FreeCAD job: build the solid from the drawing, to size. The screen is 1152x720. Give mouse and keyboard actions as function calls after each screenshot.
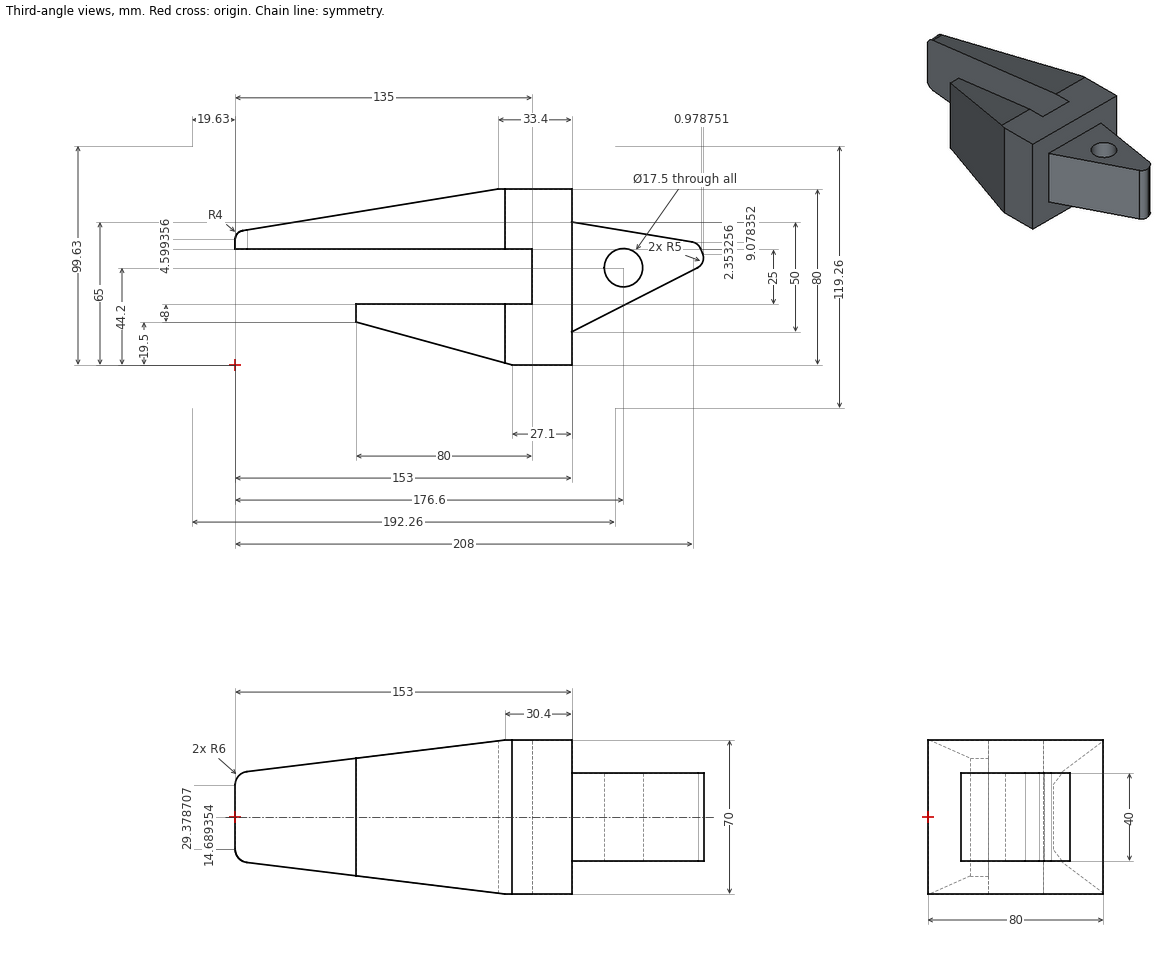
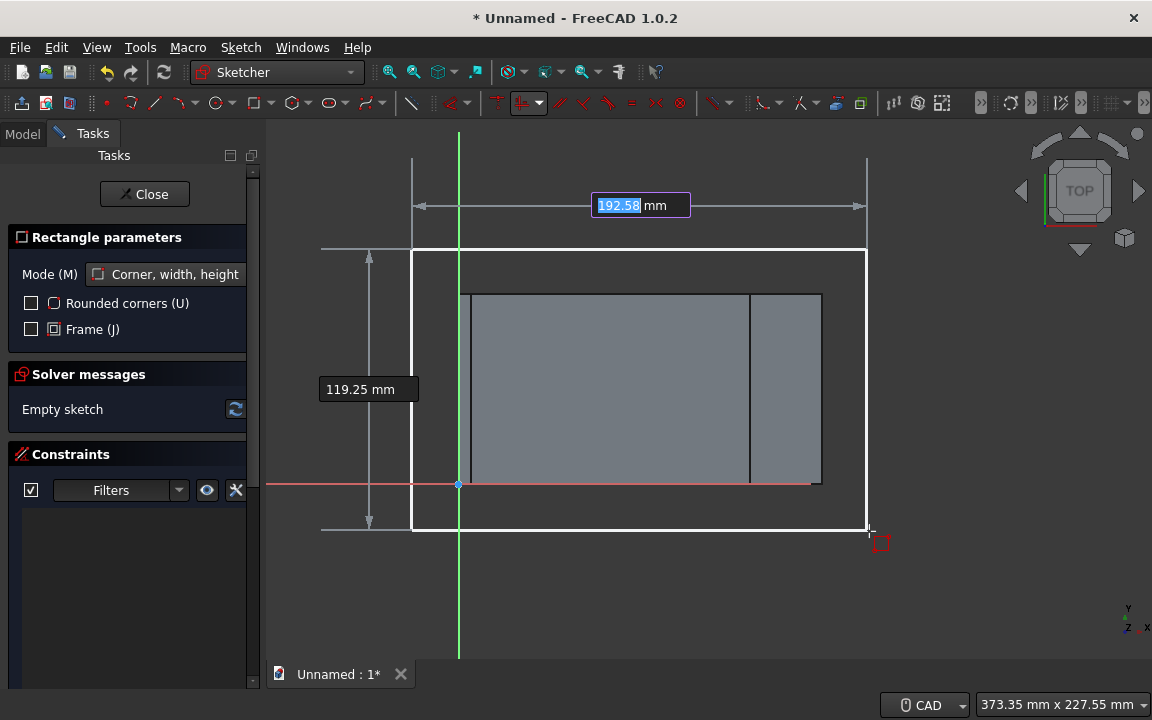
text(192.26)
key(Tab)
text(119.26)
key(Return)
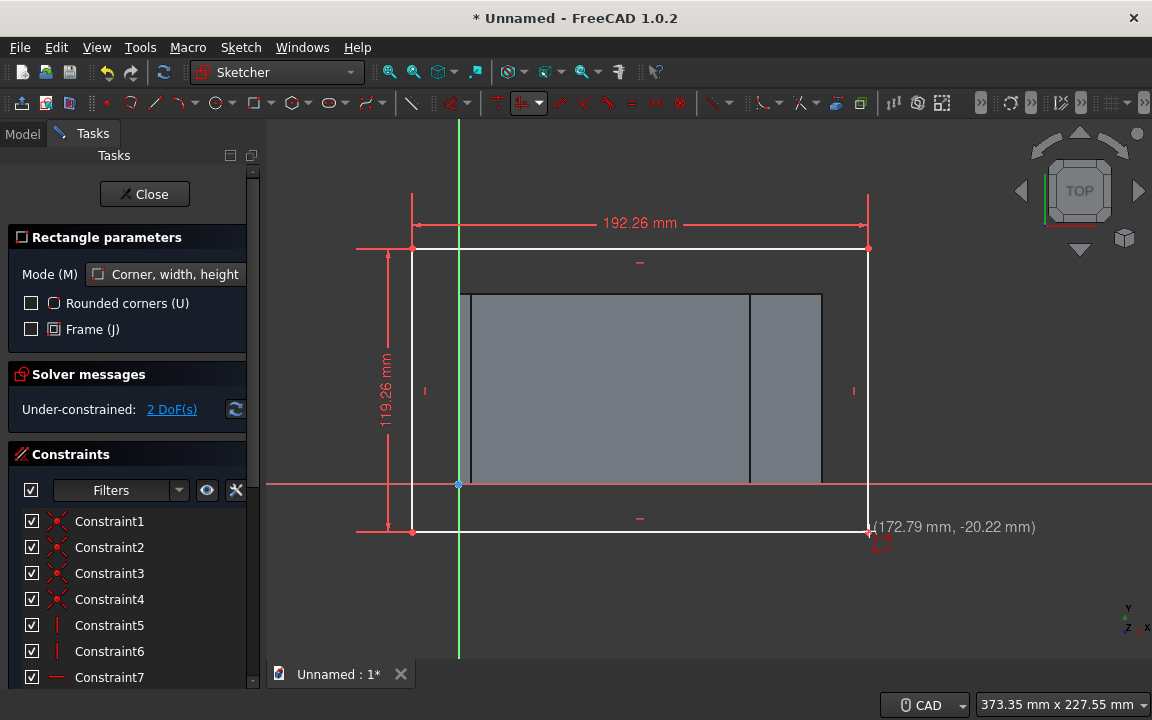
click(132, 104)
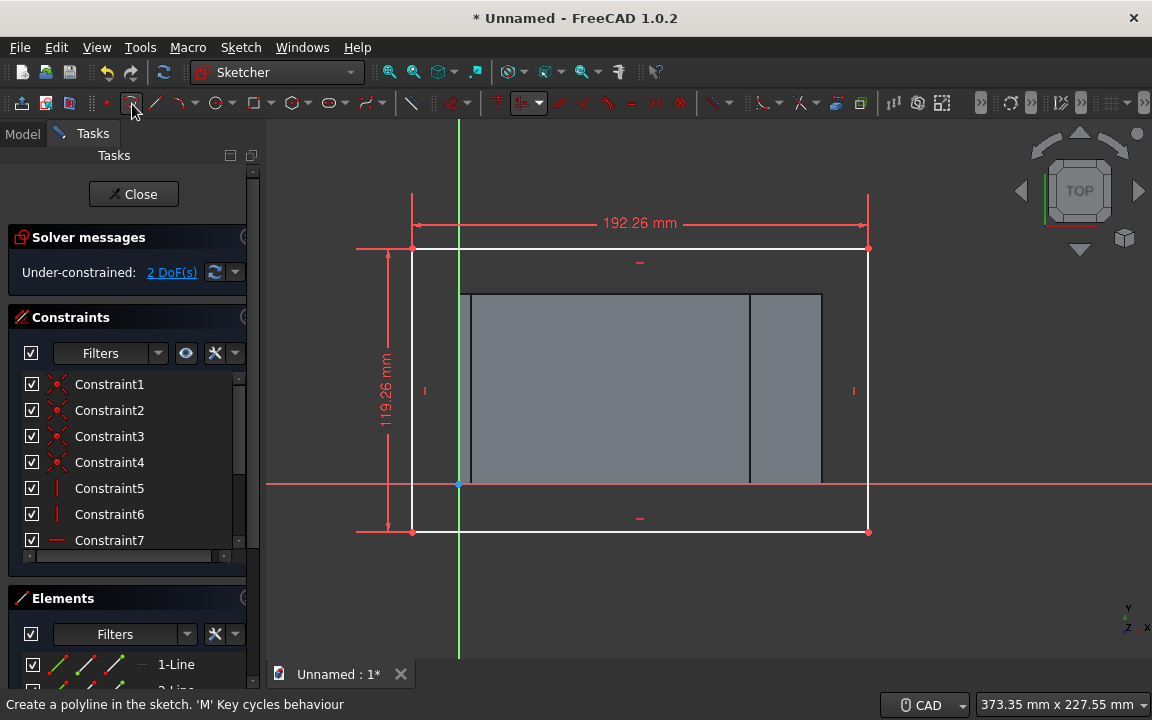
scroll(467, 339, up, 4)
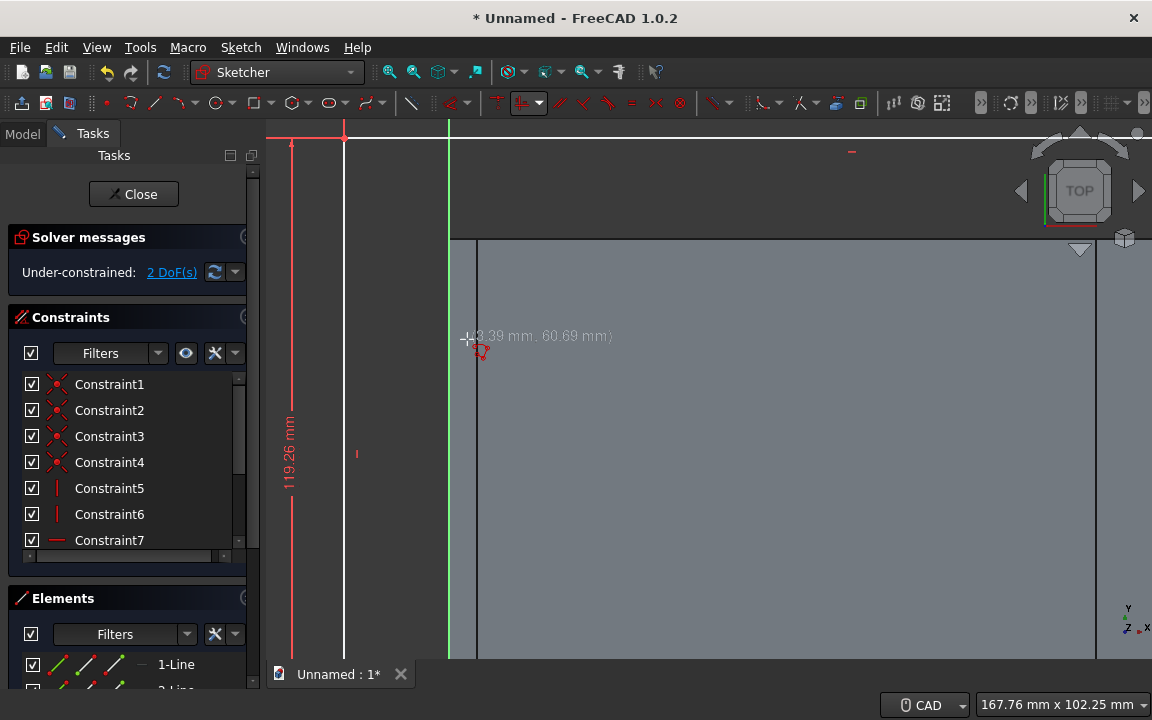
click(467, 339)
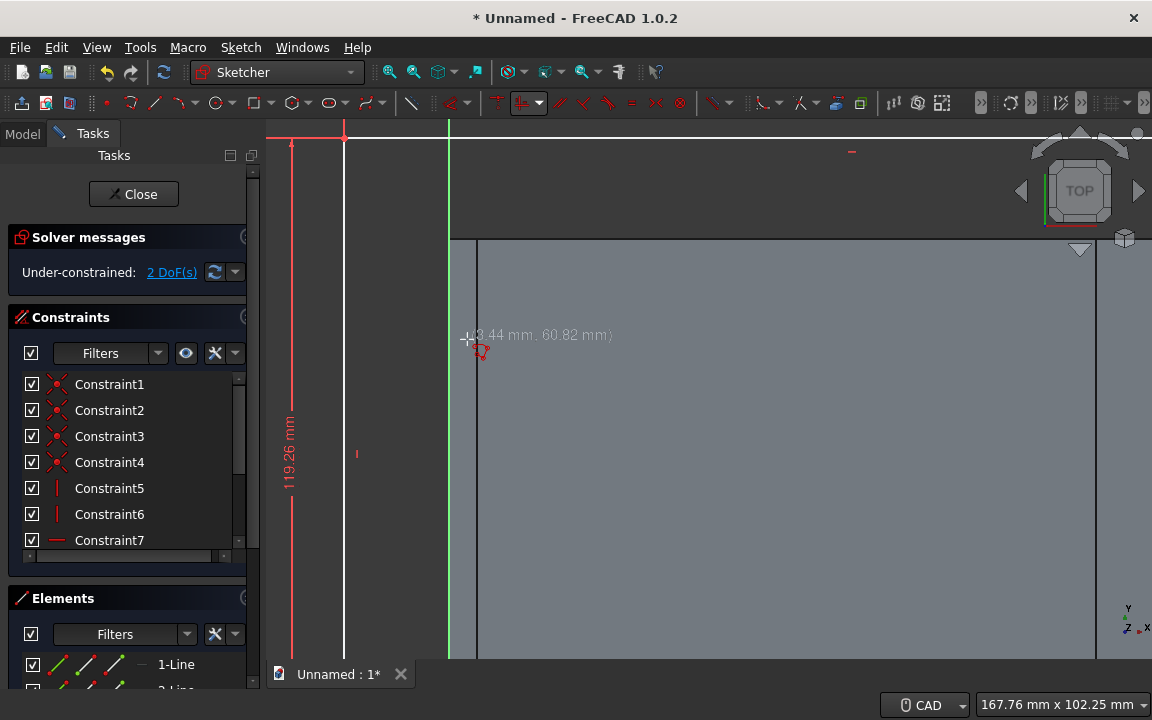
scroll(467, 339, down, 4)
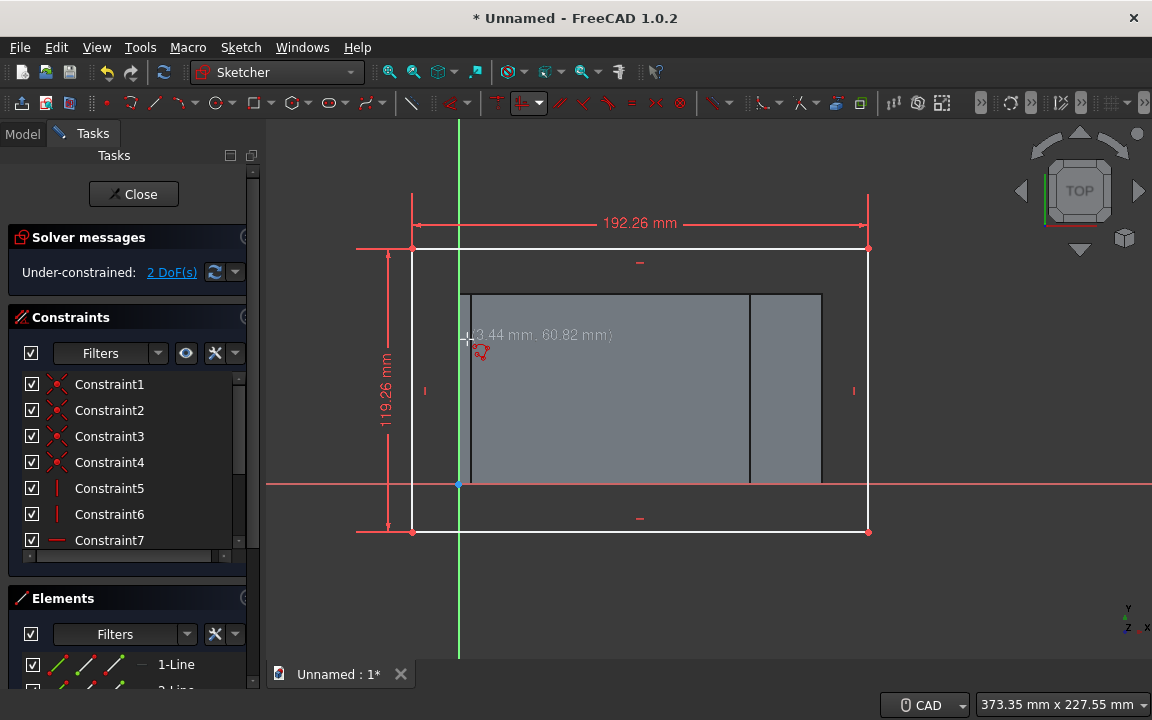
click(743, 294)
click(822, 294)
click(822, 484)
click(758, 475)
click(589, 438)
click(589, 419)
click(779, 419)
click(779, 359)
click(459, 359)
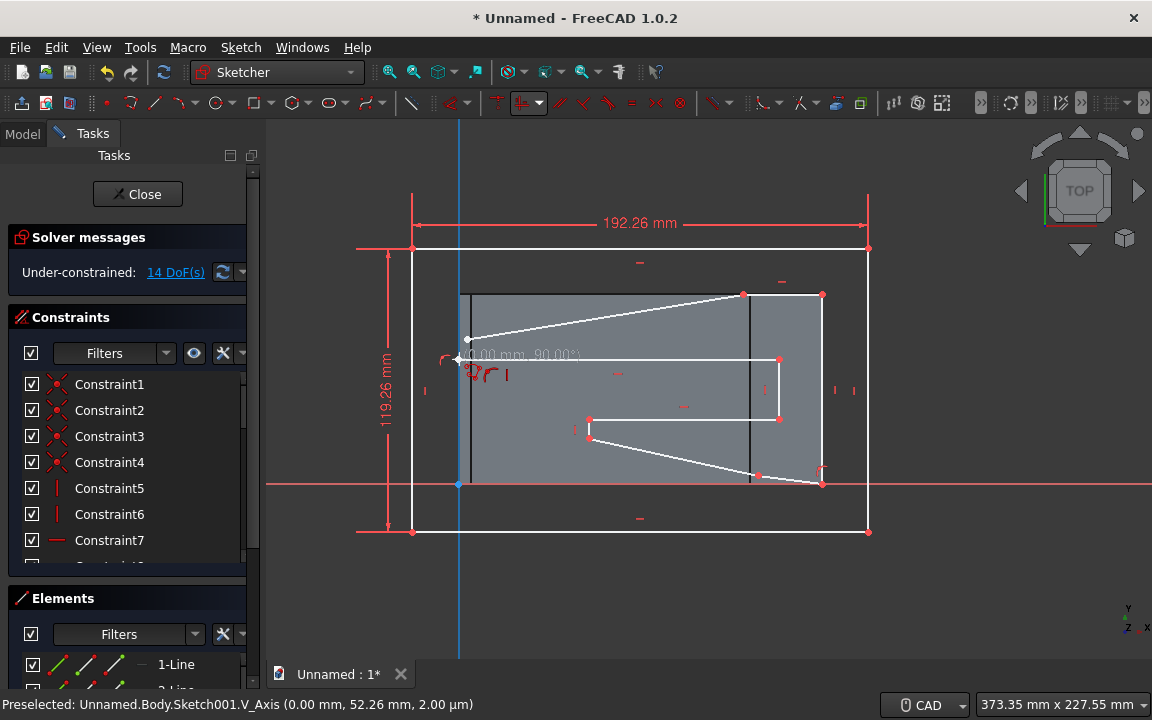
scroll(459, 349, up, 2)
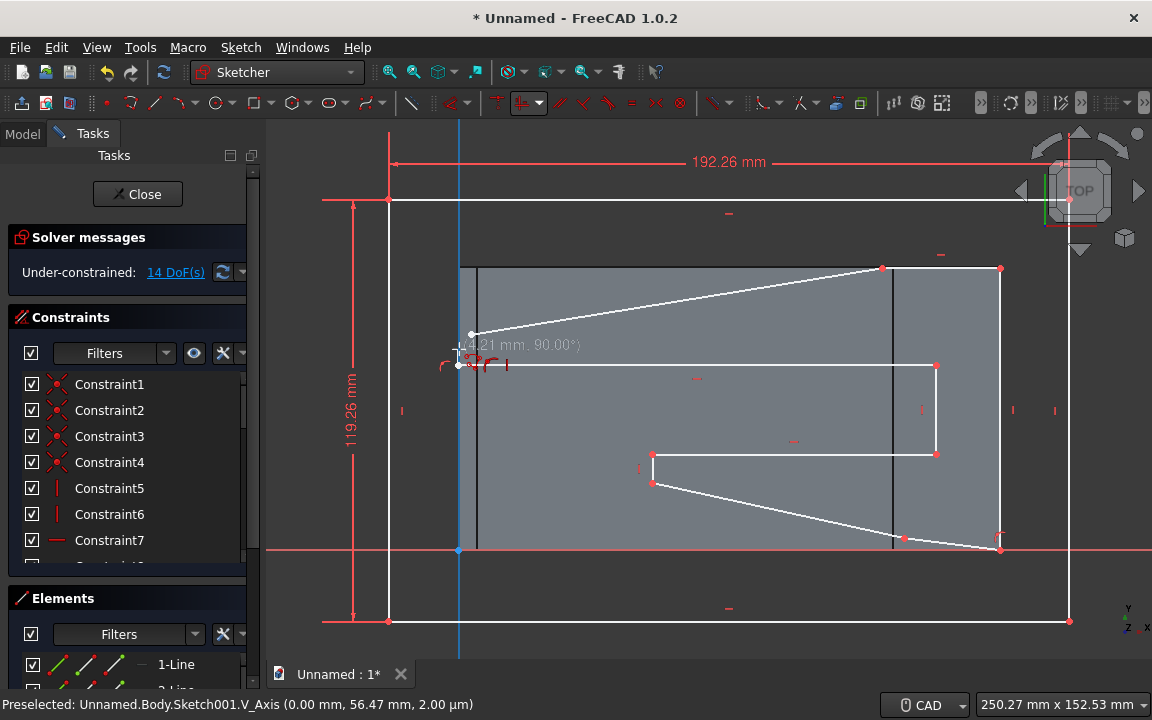
click(468, 348)
right_click(468, 348)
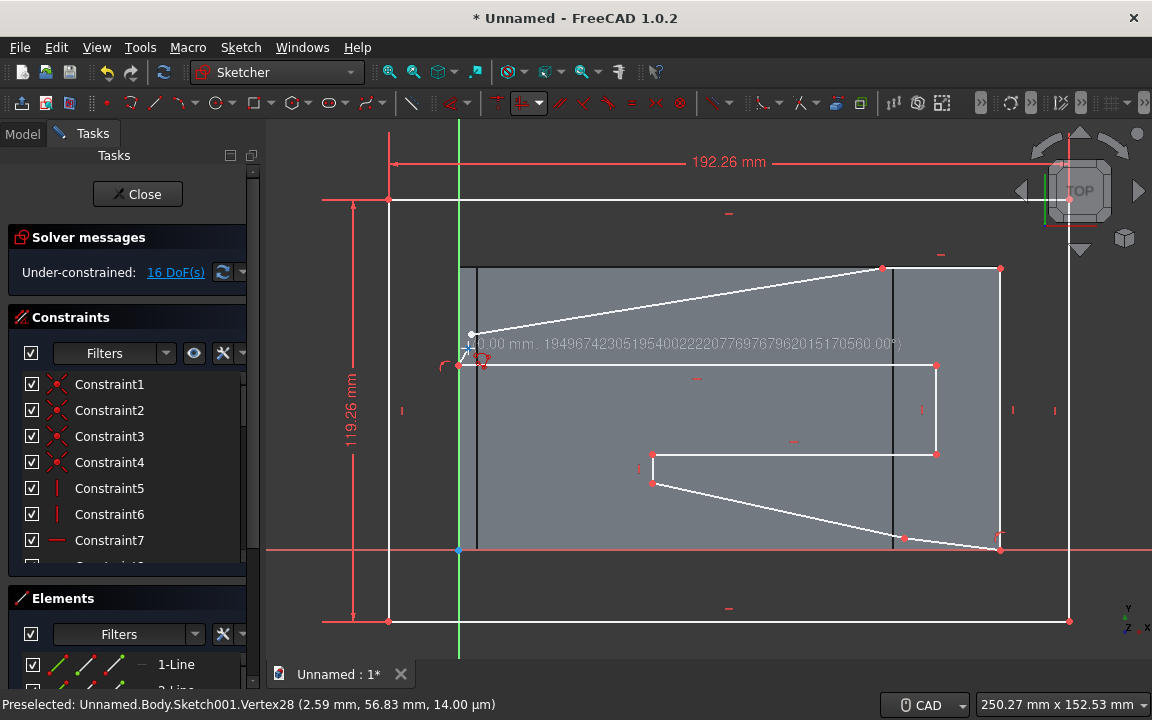
click(180, 104)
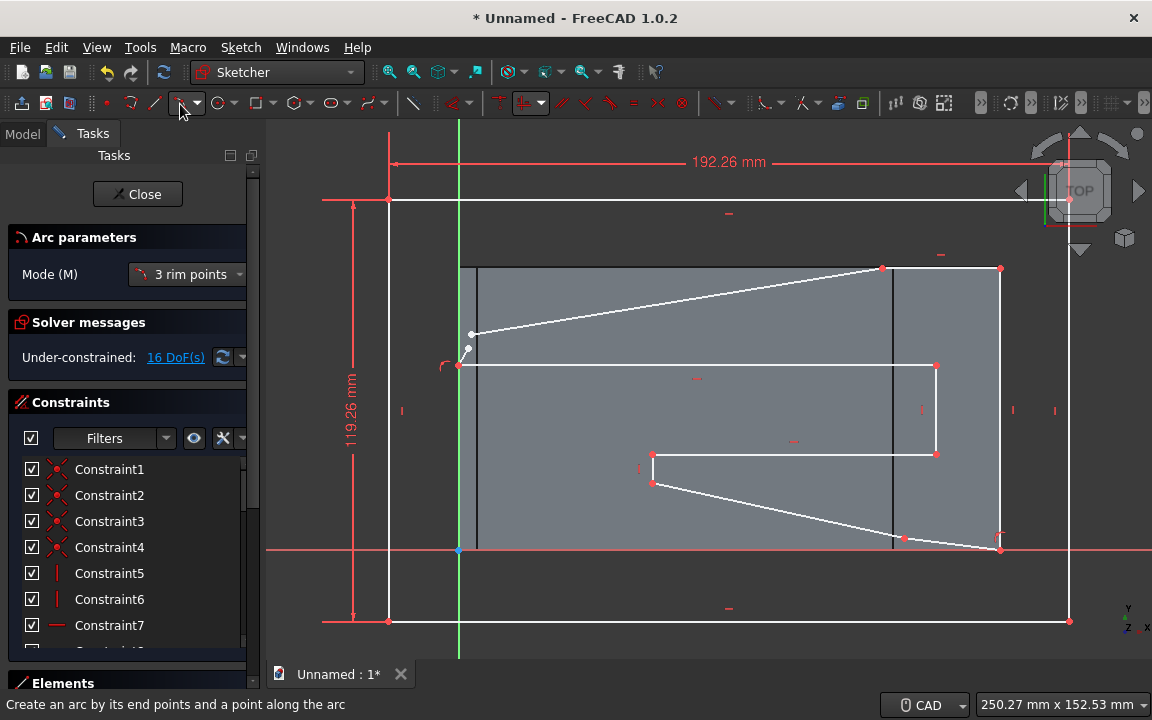
scroll(459, 348, up, 4)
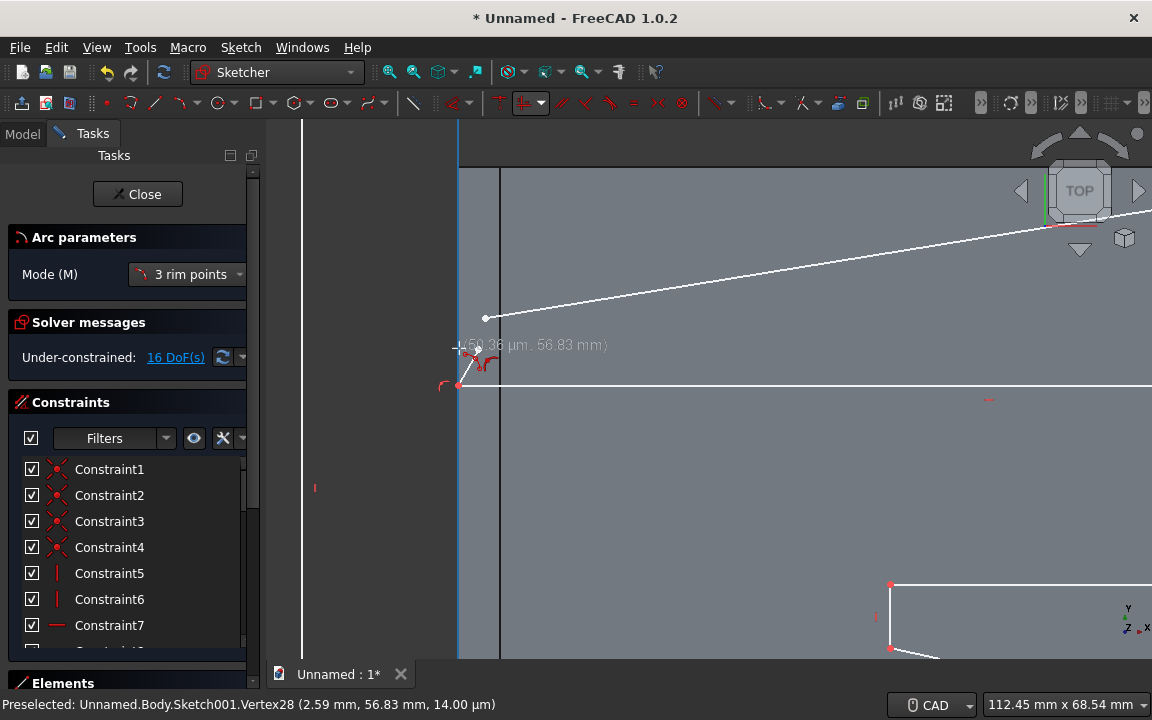
click(479, 350)
click(485, 318)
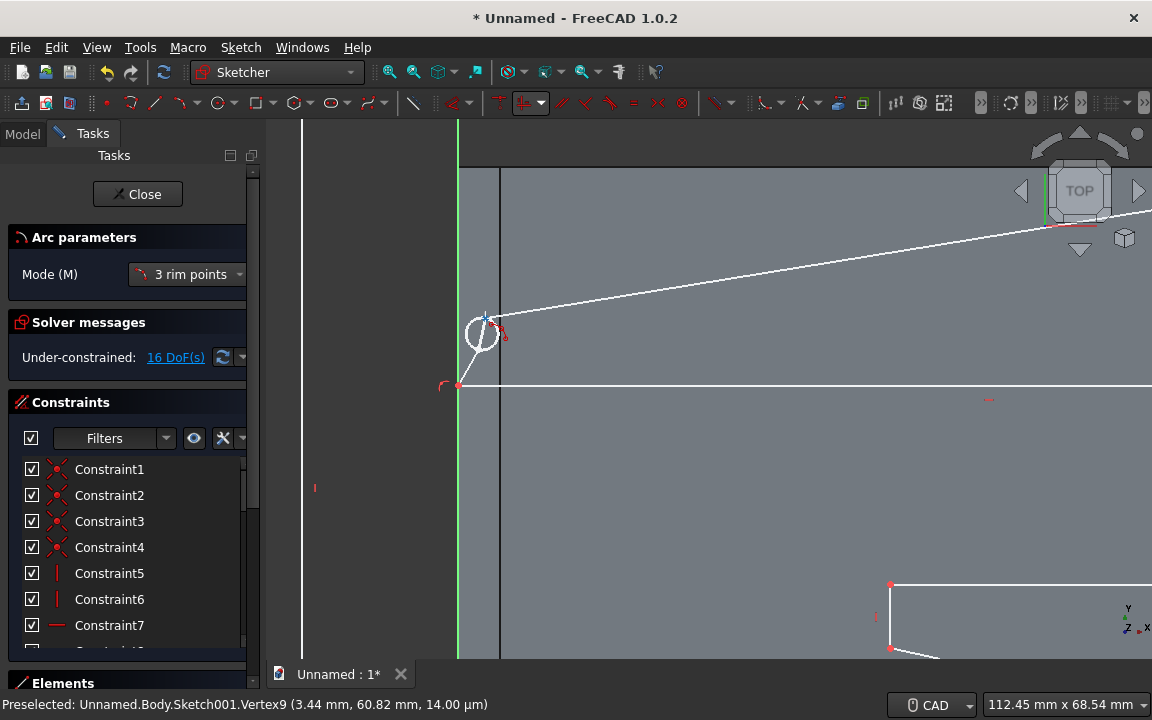
scroll(466, 327, up, 4)